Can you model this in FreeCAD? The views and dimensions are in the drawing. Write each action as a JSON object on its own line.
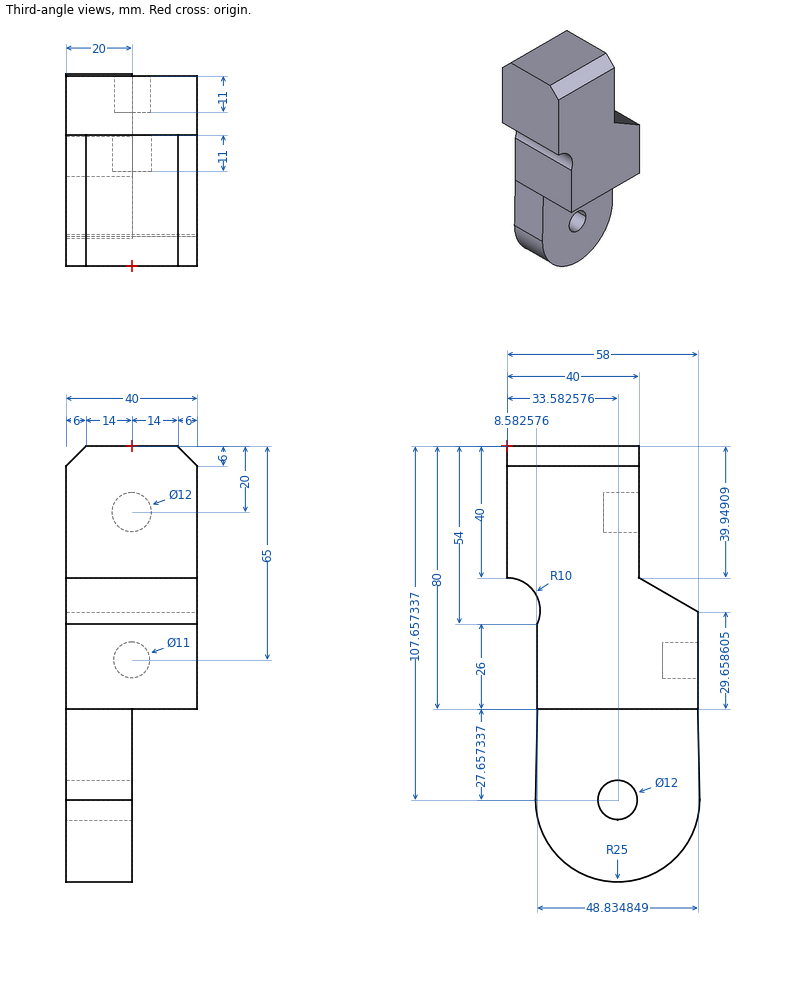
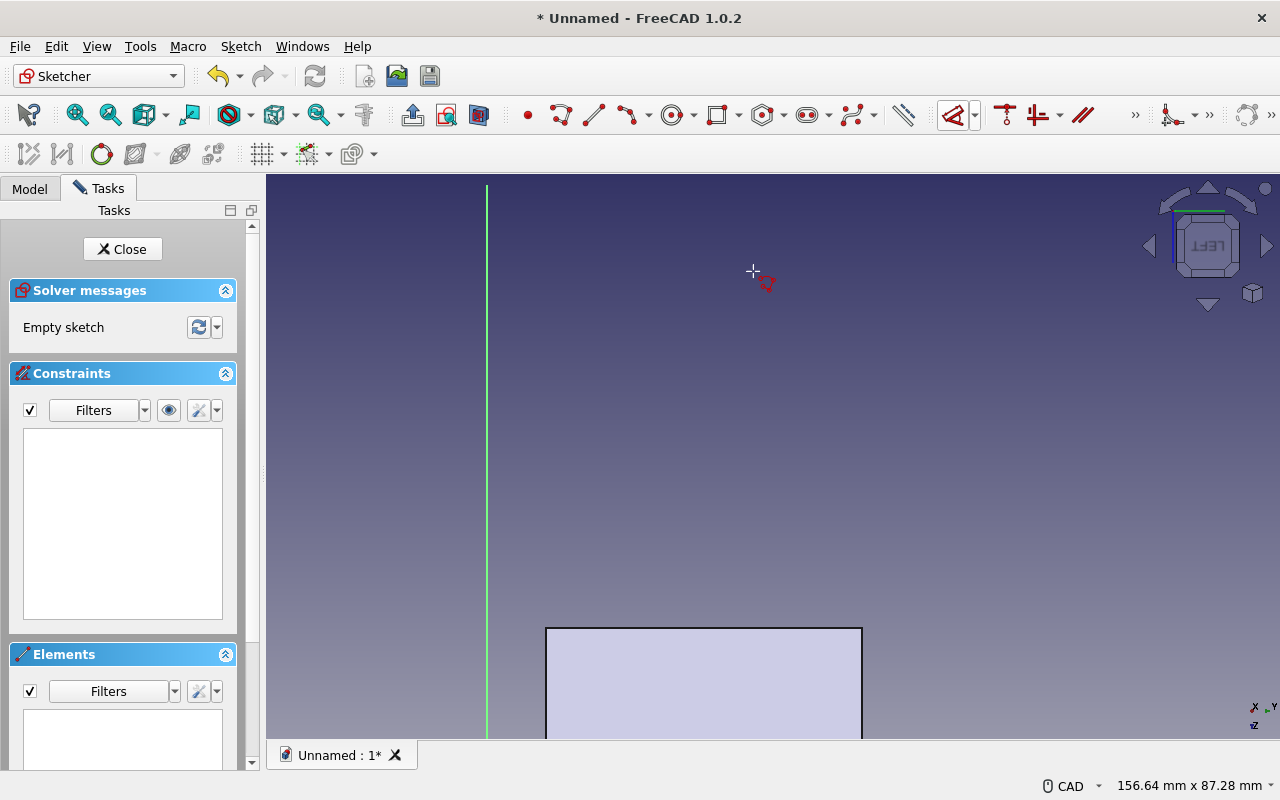
{"action": "left_click", "coordinate": [542, 449]}
{"action": "left_click", "coordinate": [552, 628]}
{"action": "left_click", "coordinate": [862, 628]}
{"action": "left_click", "coordinate": [872, 449]}
{"action": "right_click", "coordinate": [872, 449]}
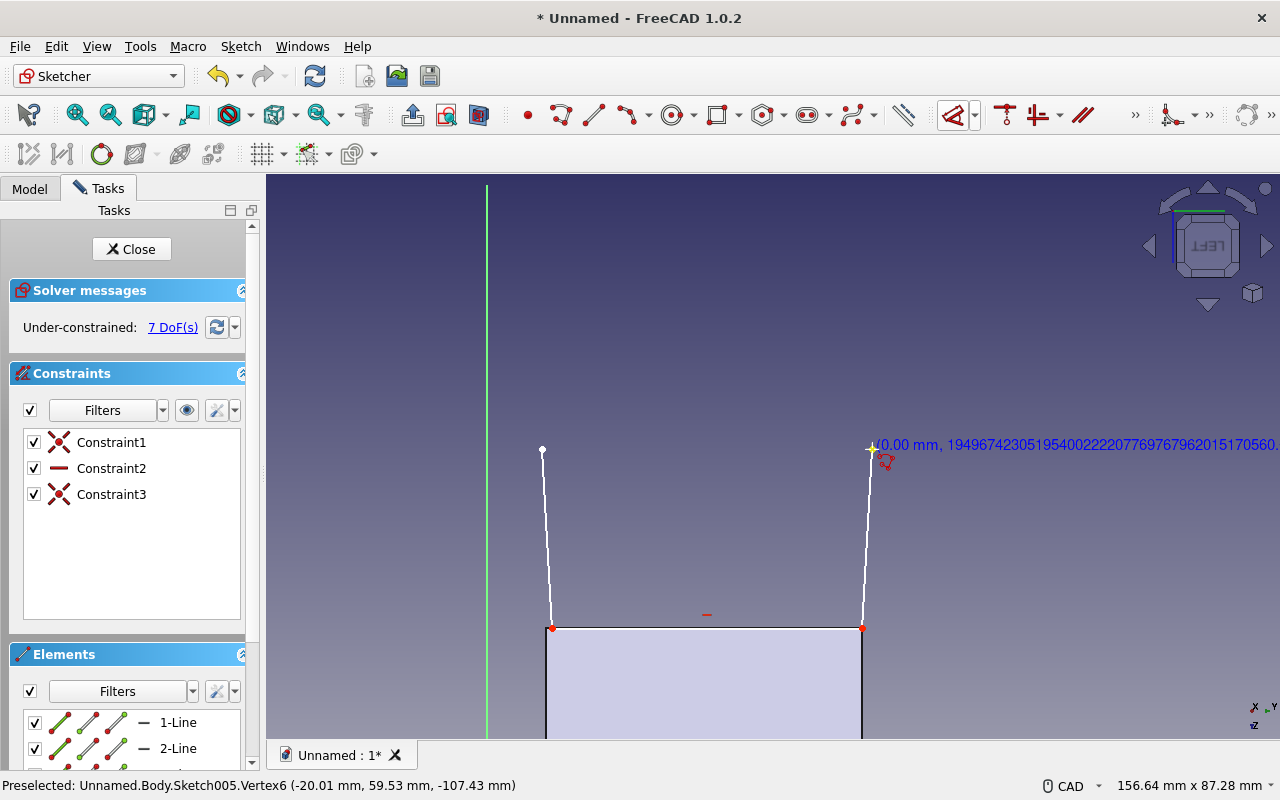
{"action": "left_click", "coordinate": [626, 116]}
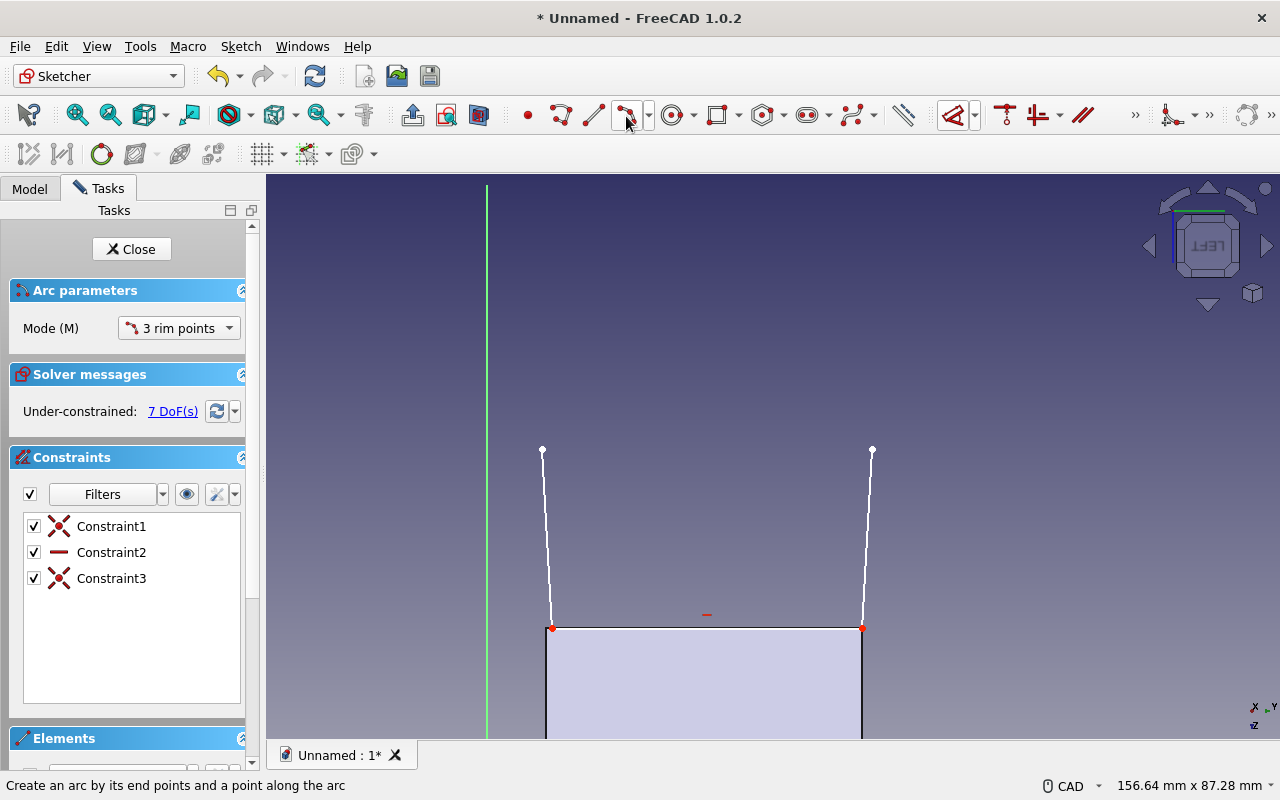
{"action": "left_click", "coordinate": [872, 450]}
{"action": "left_click", "coordinate": [542, 450]}
{"action": "left_click", "coordinate": [704, 287]}
{"action": "key", "text": "Escape"}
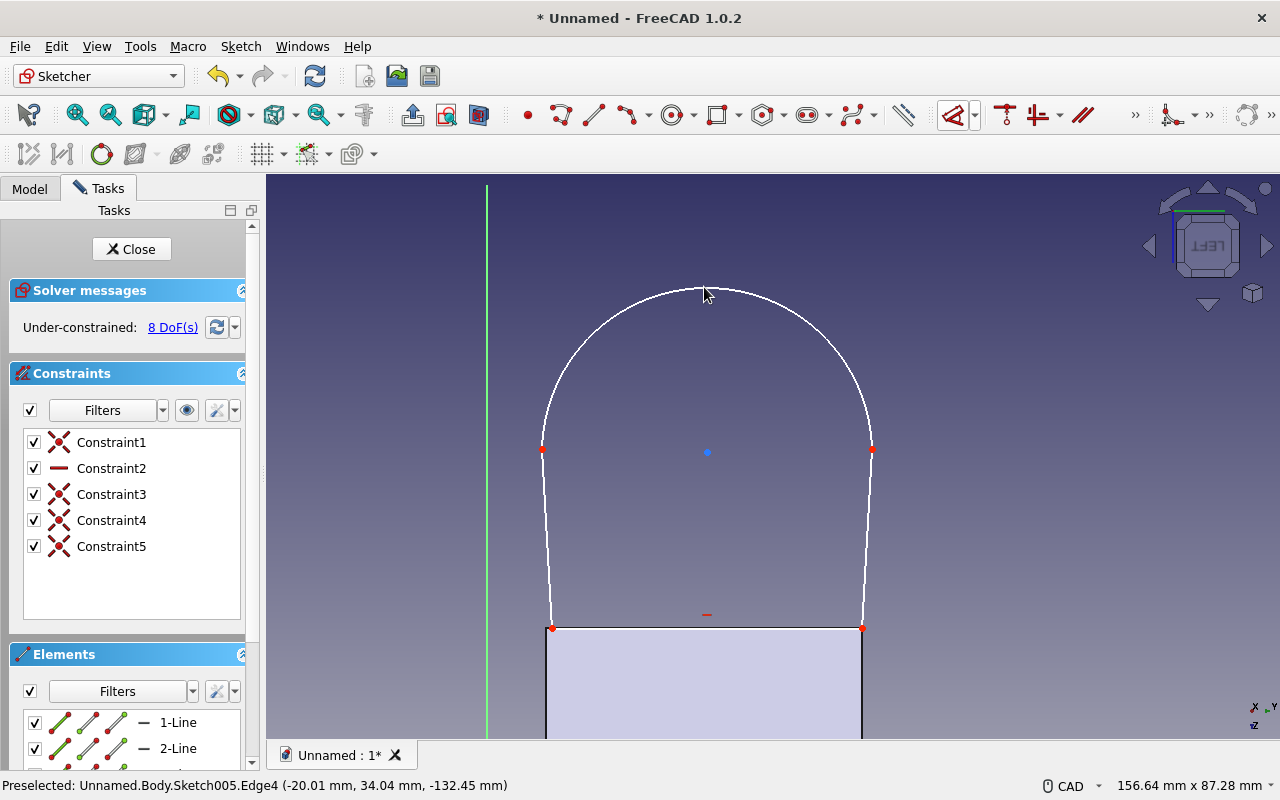
{"action": "left_click", "coordinate": [803, 319]}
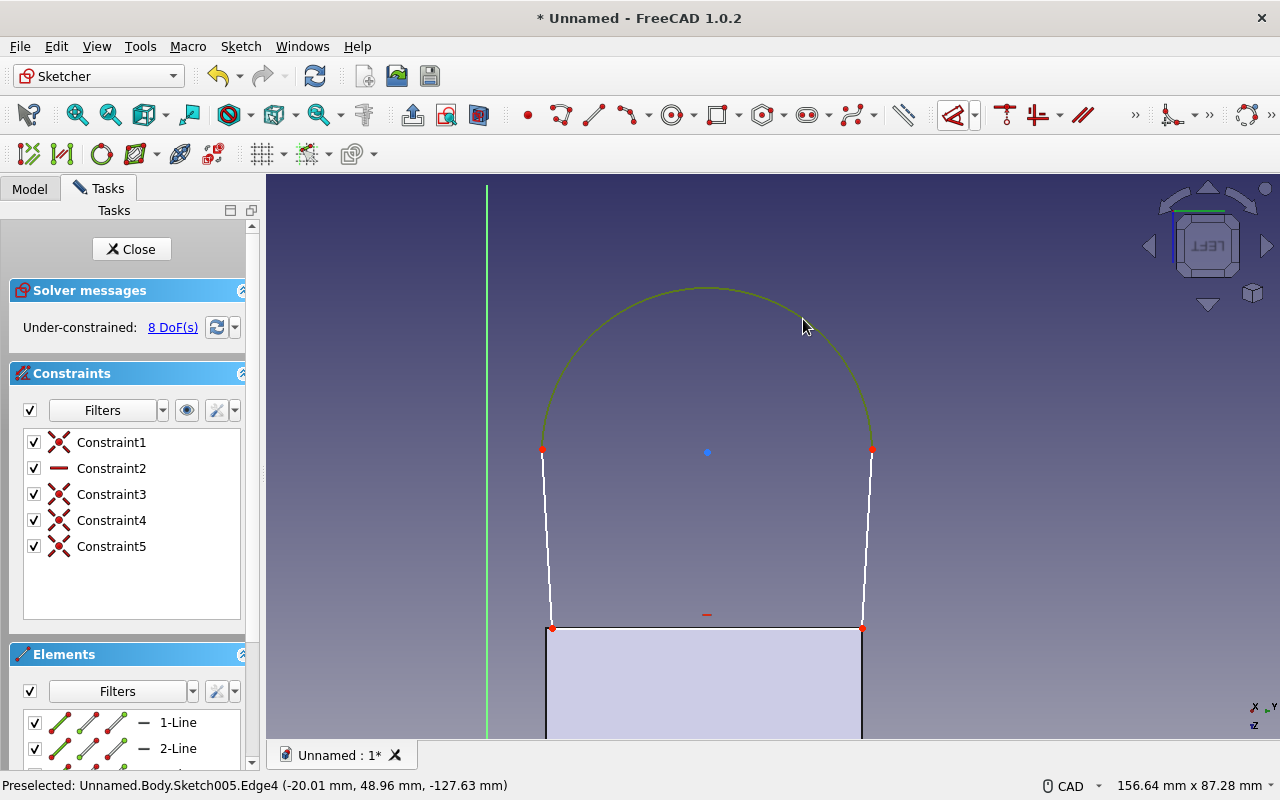
{"action": "key", "text": "k r"}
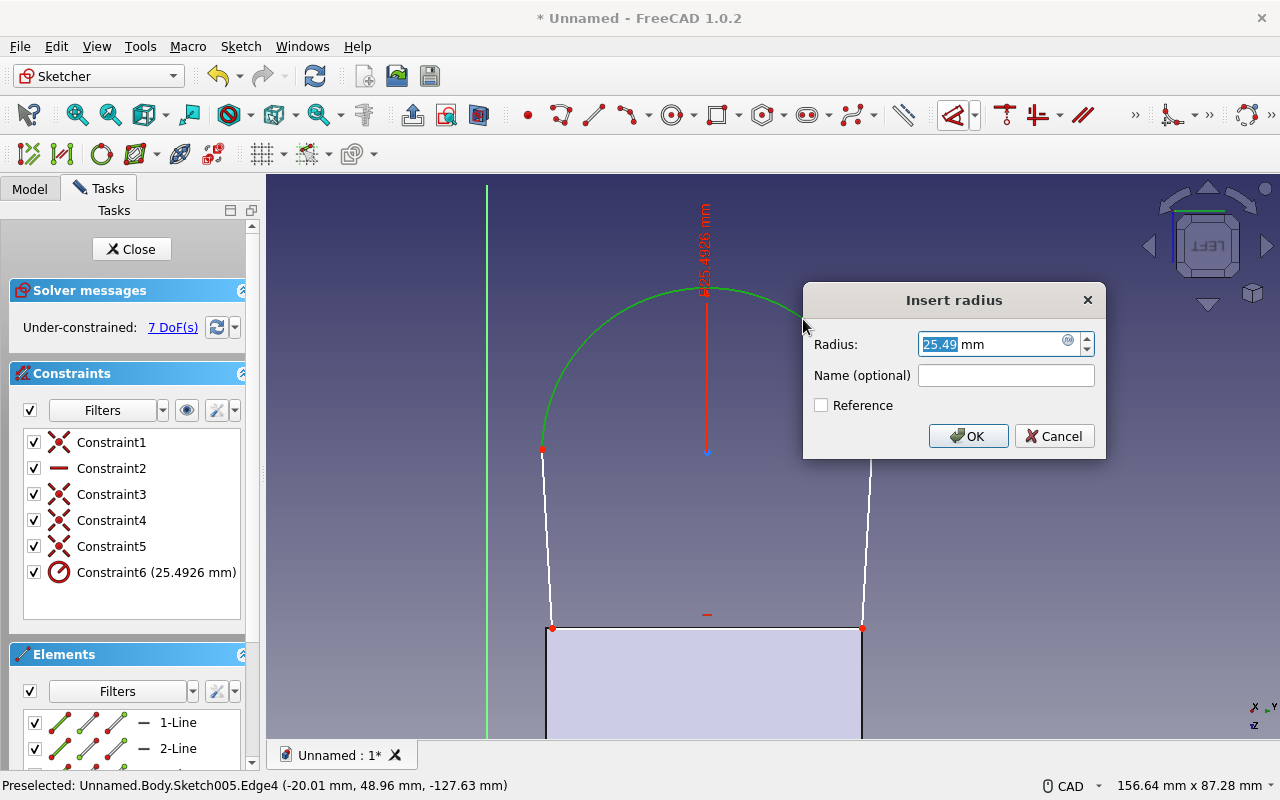
{"action": "type", "text": "25"}
{"action": "key", "text": "Return"}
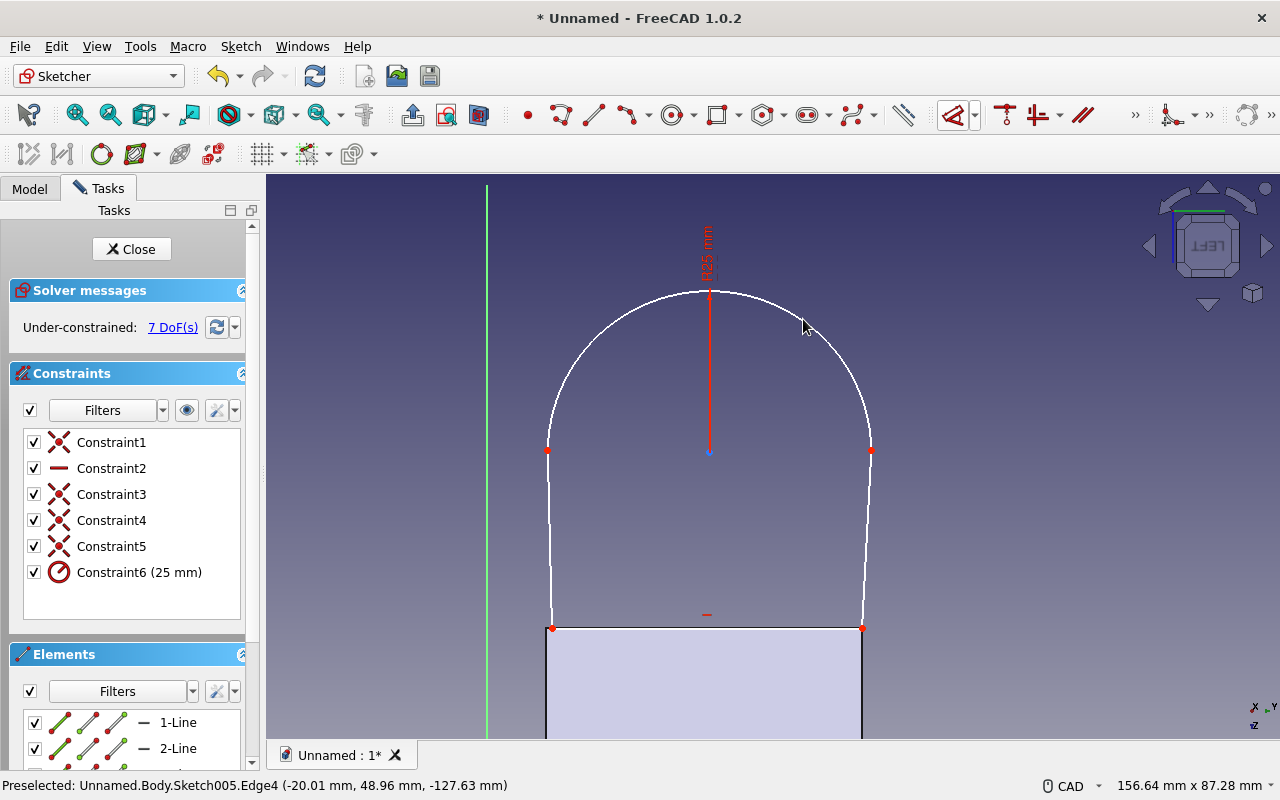
{"action": "left_click", "coordinate": [552, 629]}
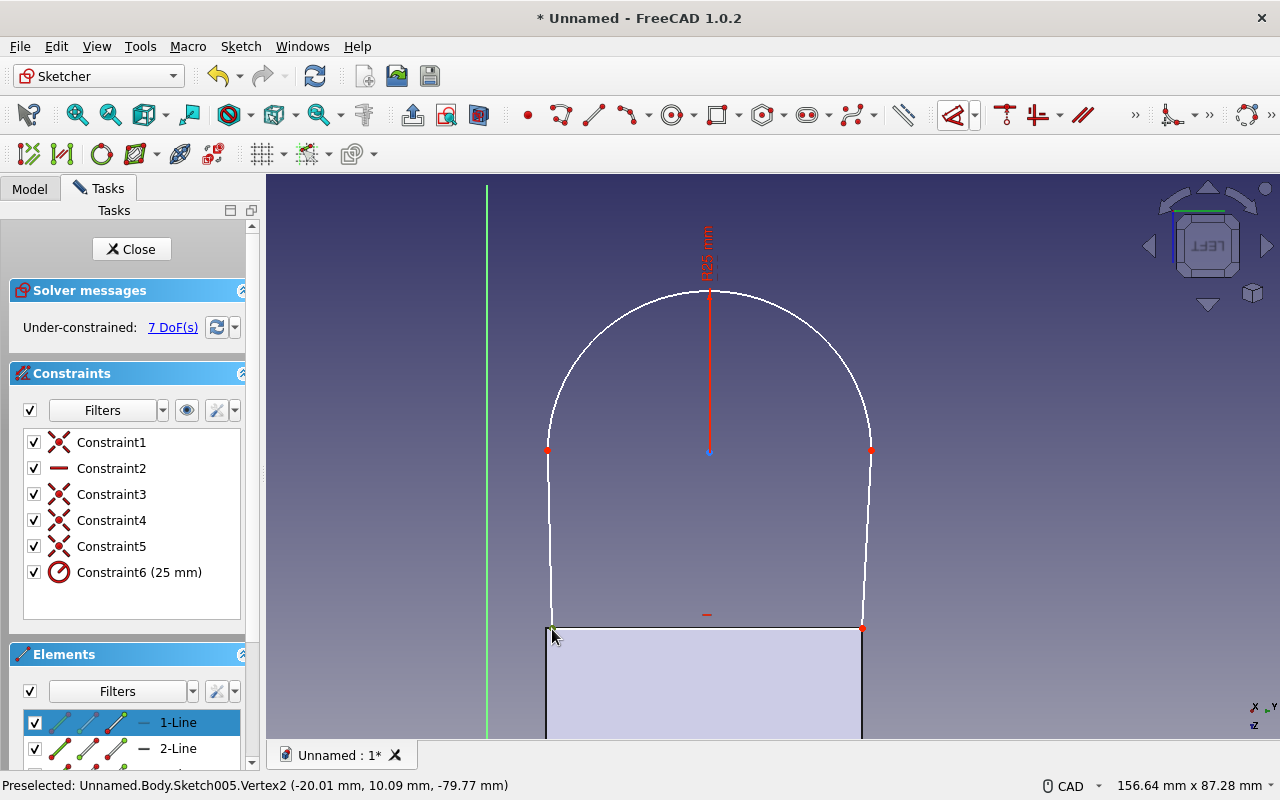
{"action": "left_click", "coordinate": [974, 116]}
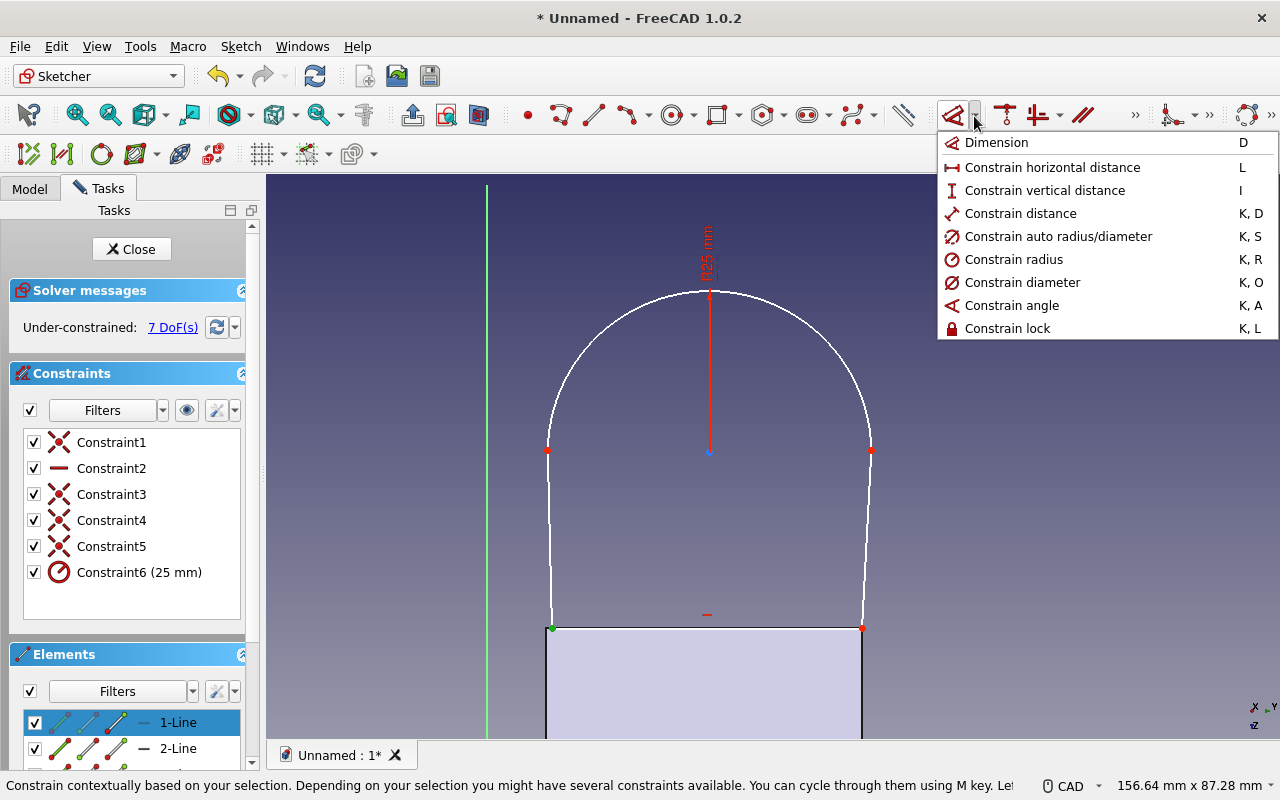
{"action": "left_click", "coordinate": [1108, 190]}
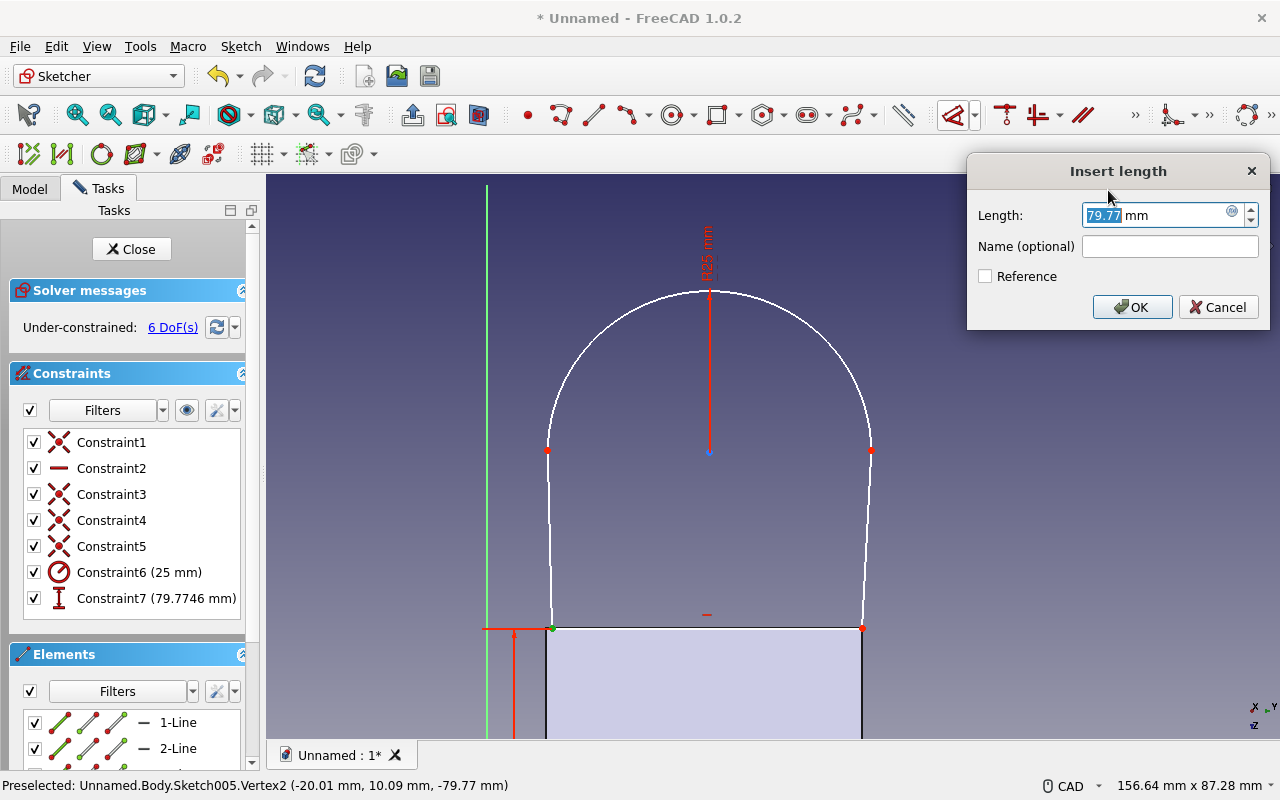
{"action": "type", "text": "80"}
{"action": "key", "text": "Return"}